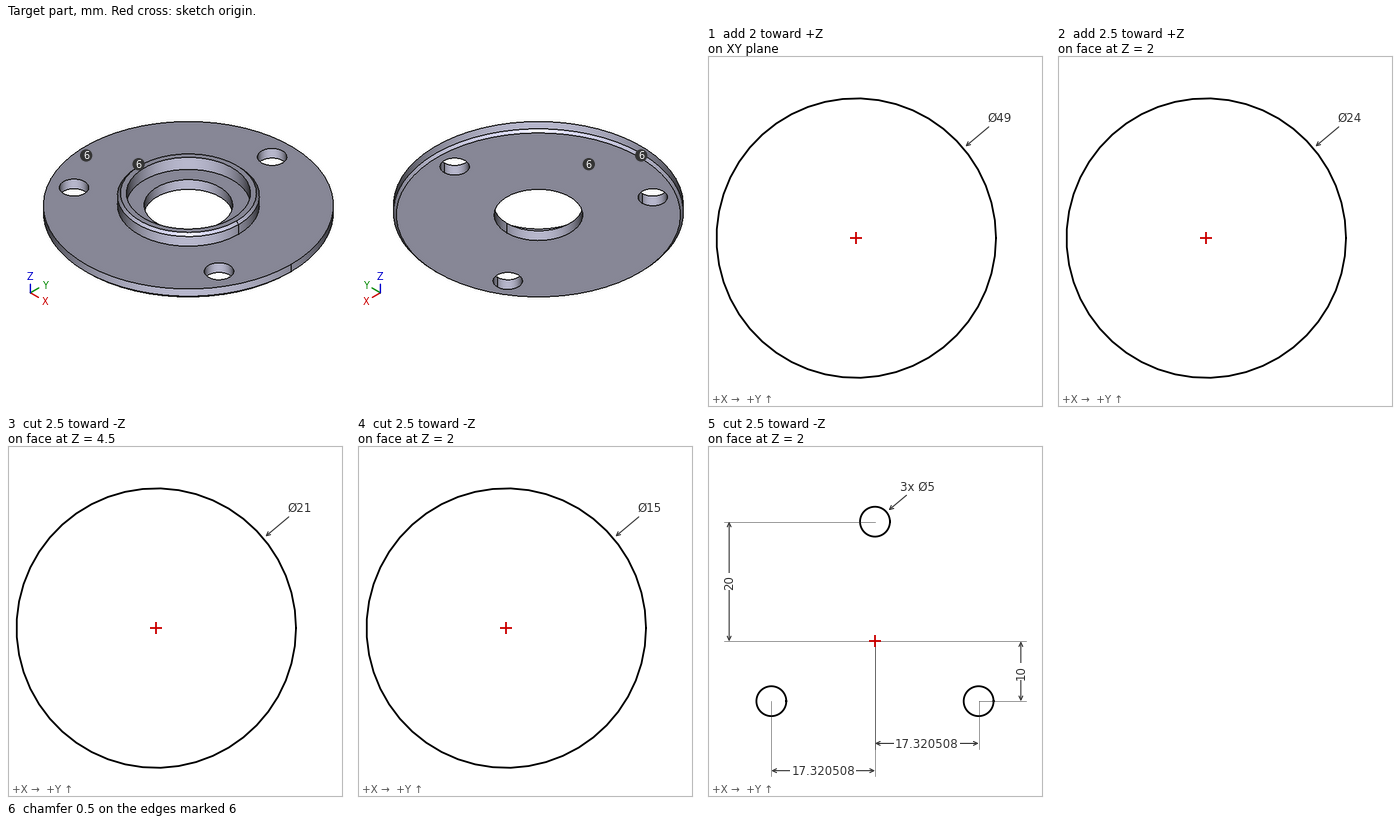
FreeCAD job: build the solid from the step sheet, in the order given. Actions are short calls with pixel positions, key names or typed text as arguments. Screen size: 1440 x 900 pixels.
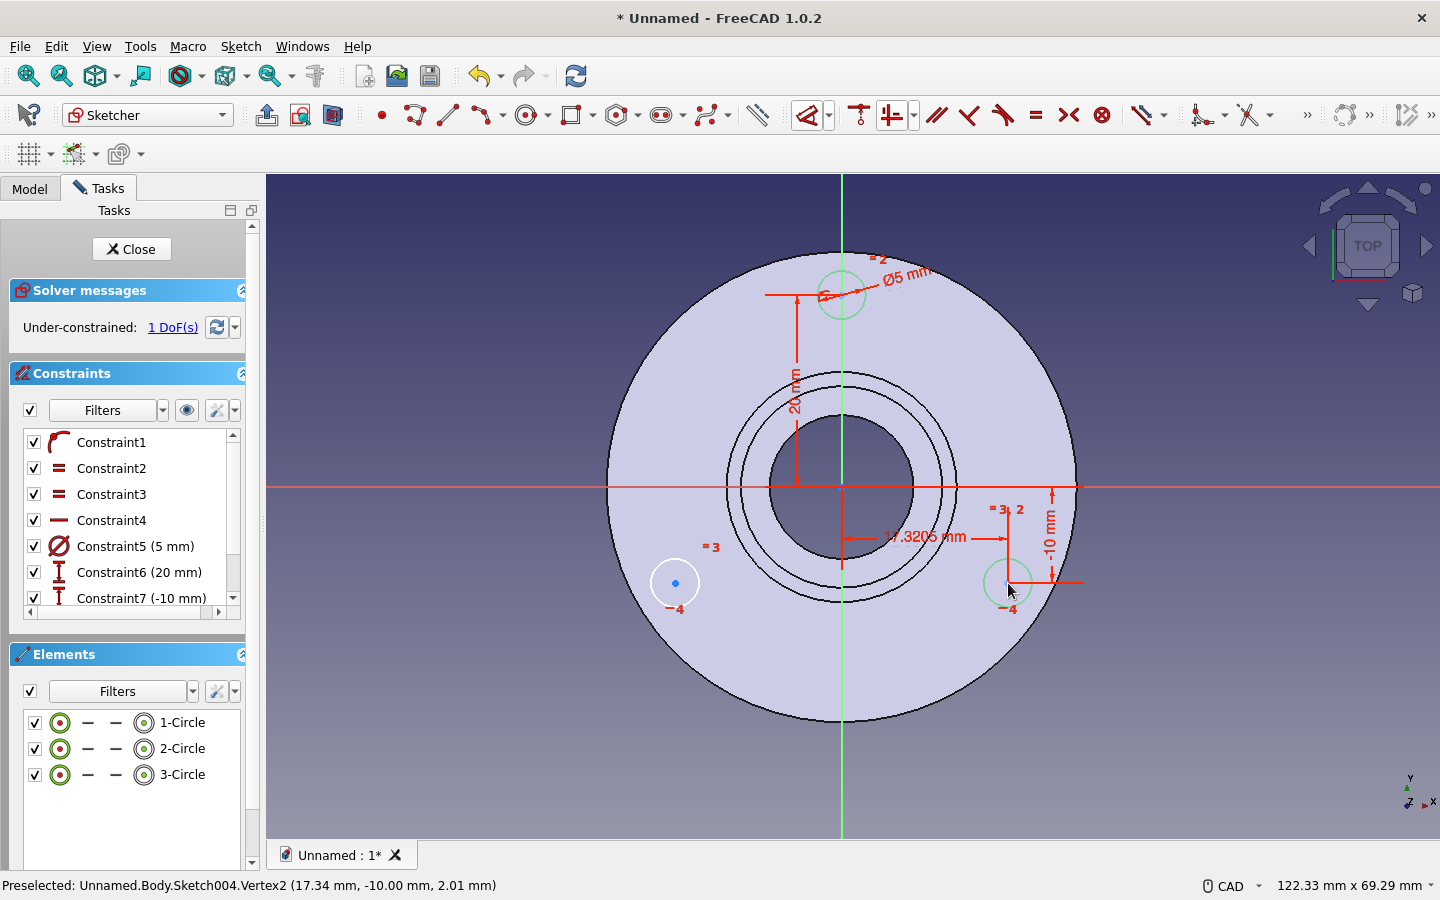
click(675, 583)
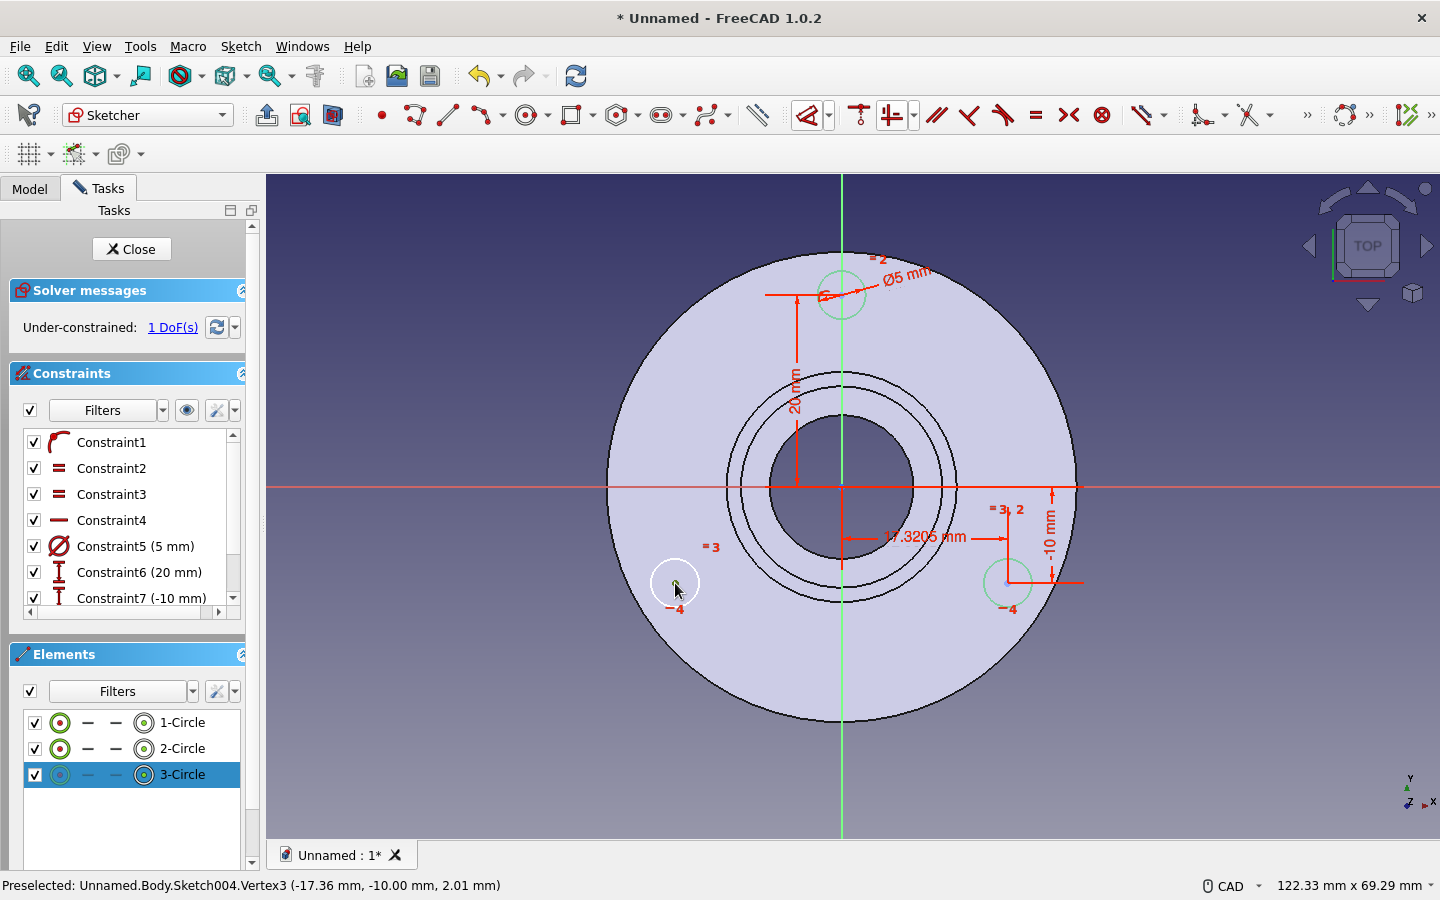
click(828, 116)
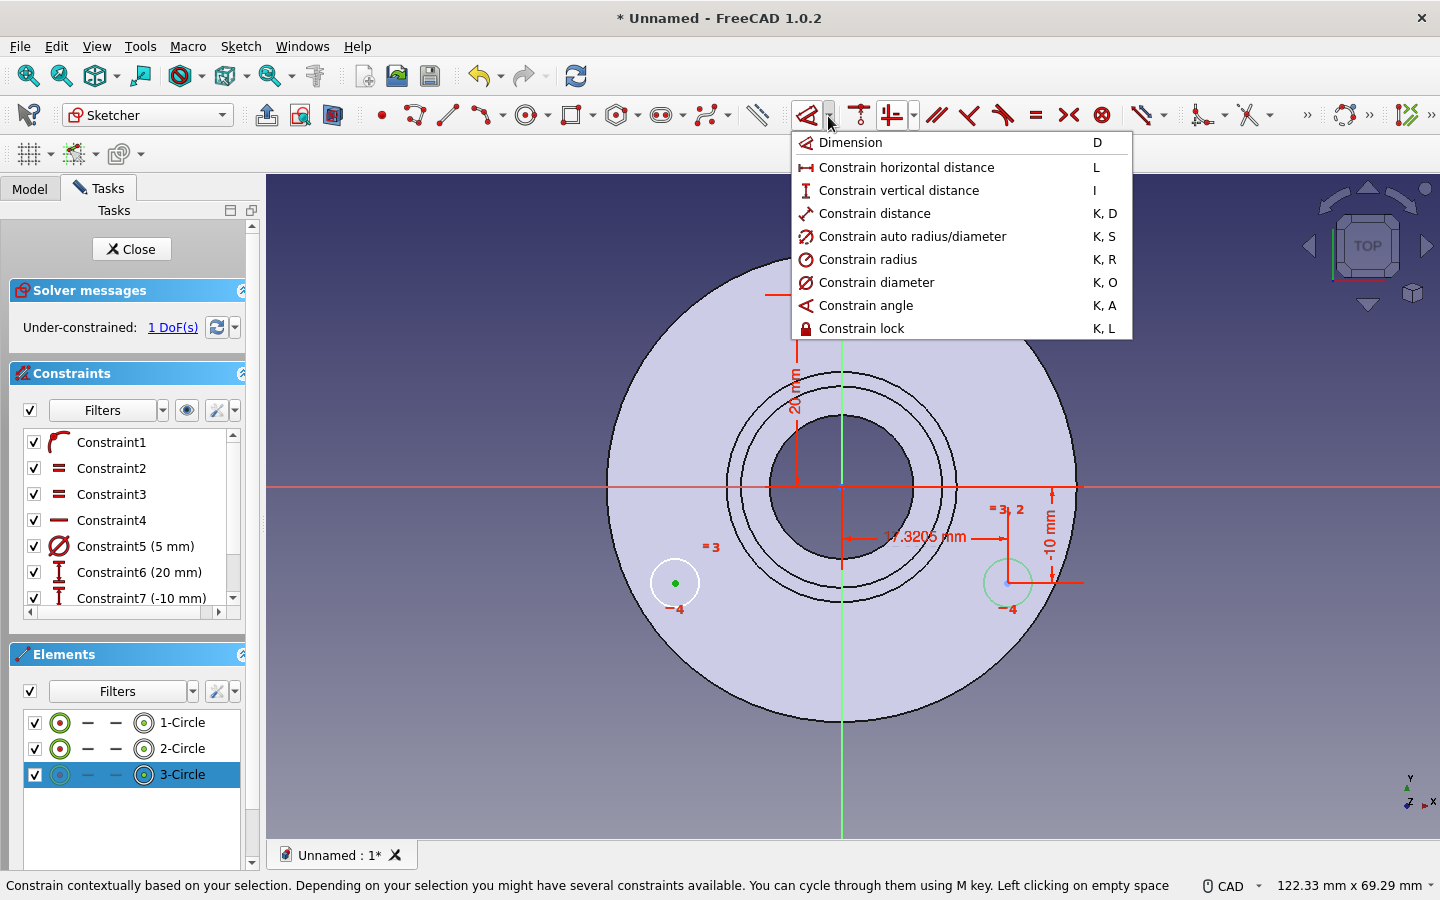
click(962, 168)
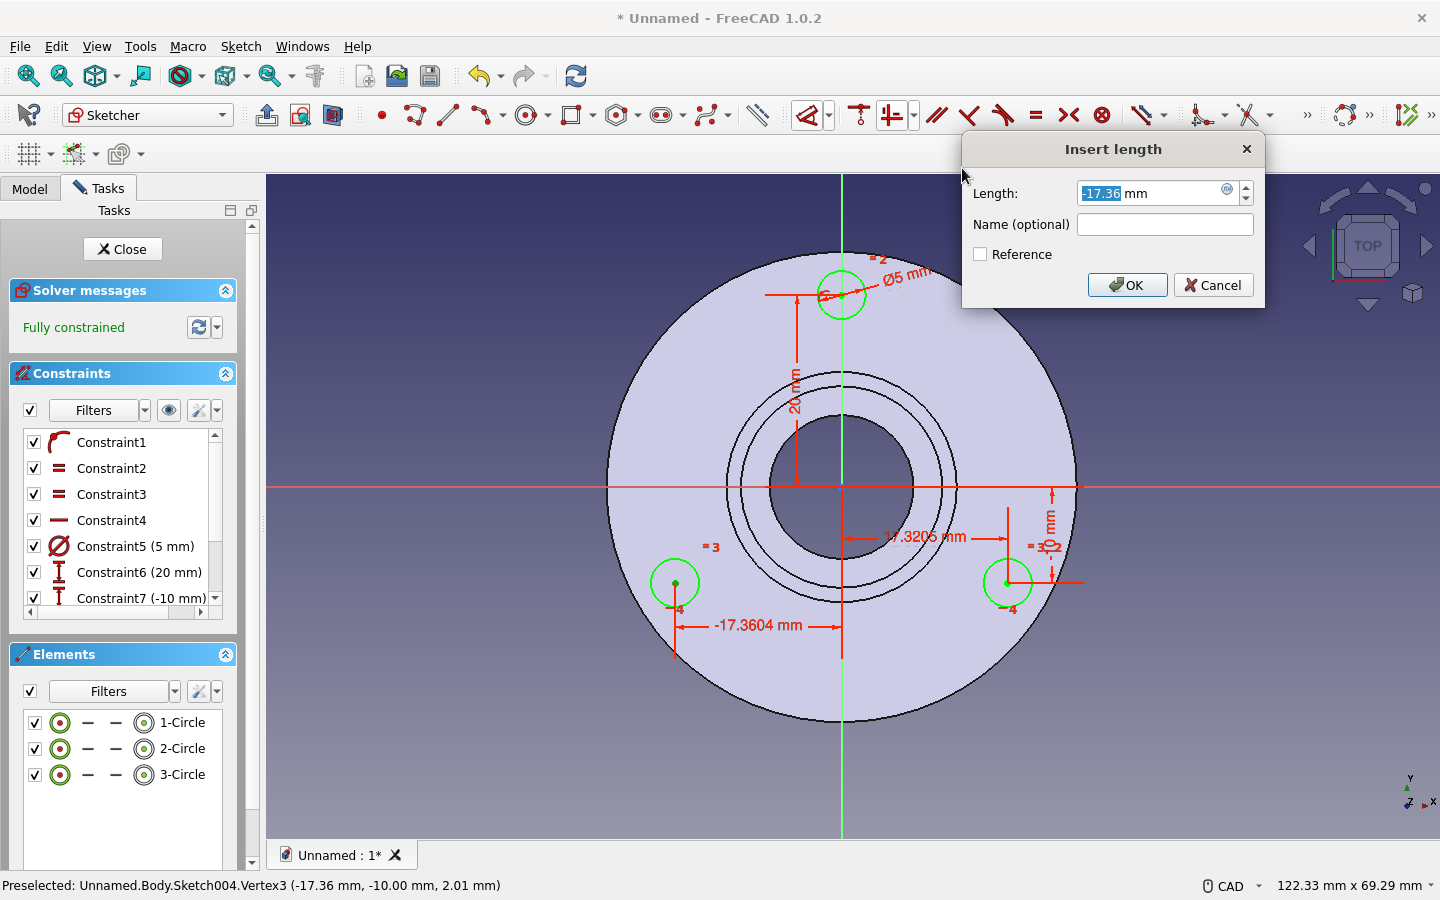
text(-17.320508)
key(Return)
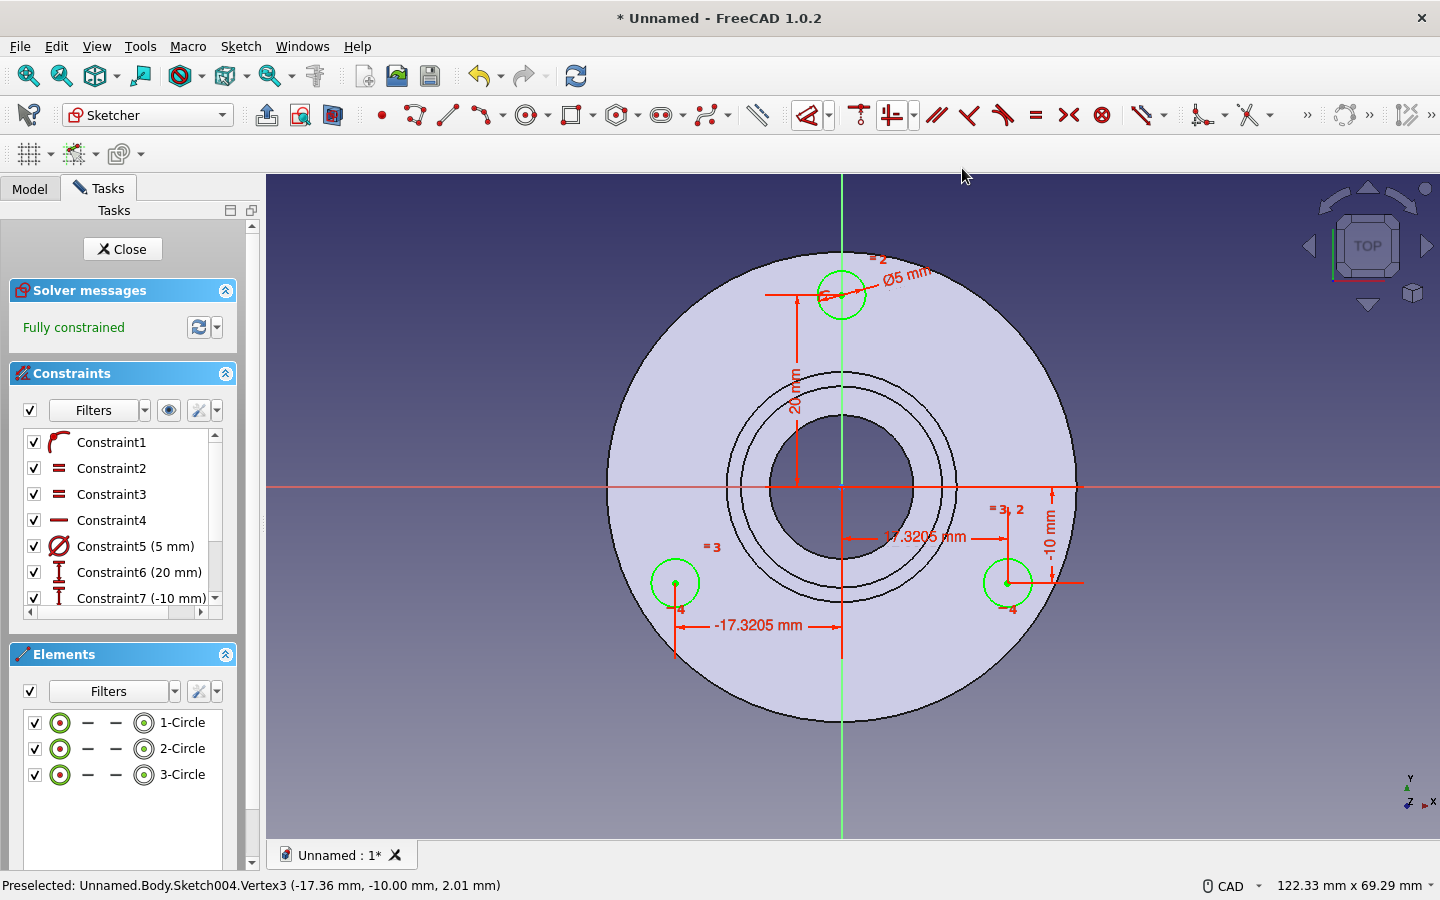
click(123, 249)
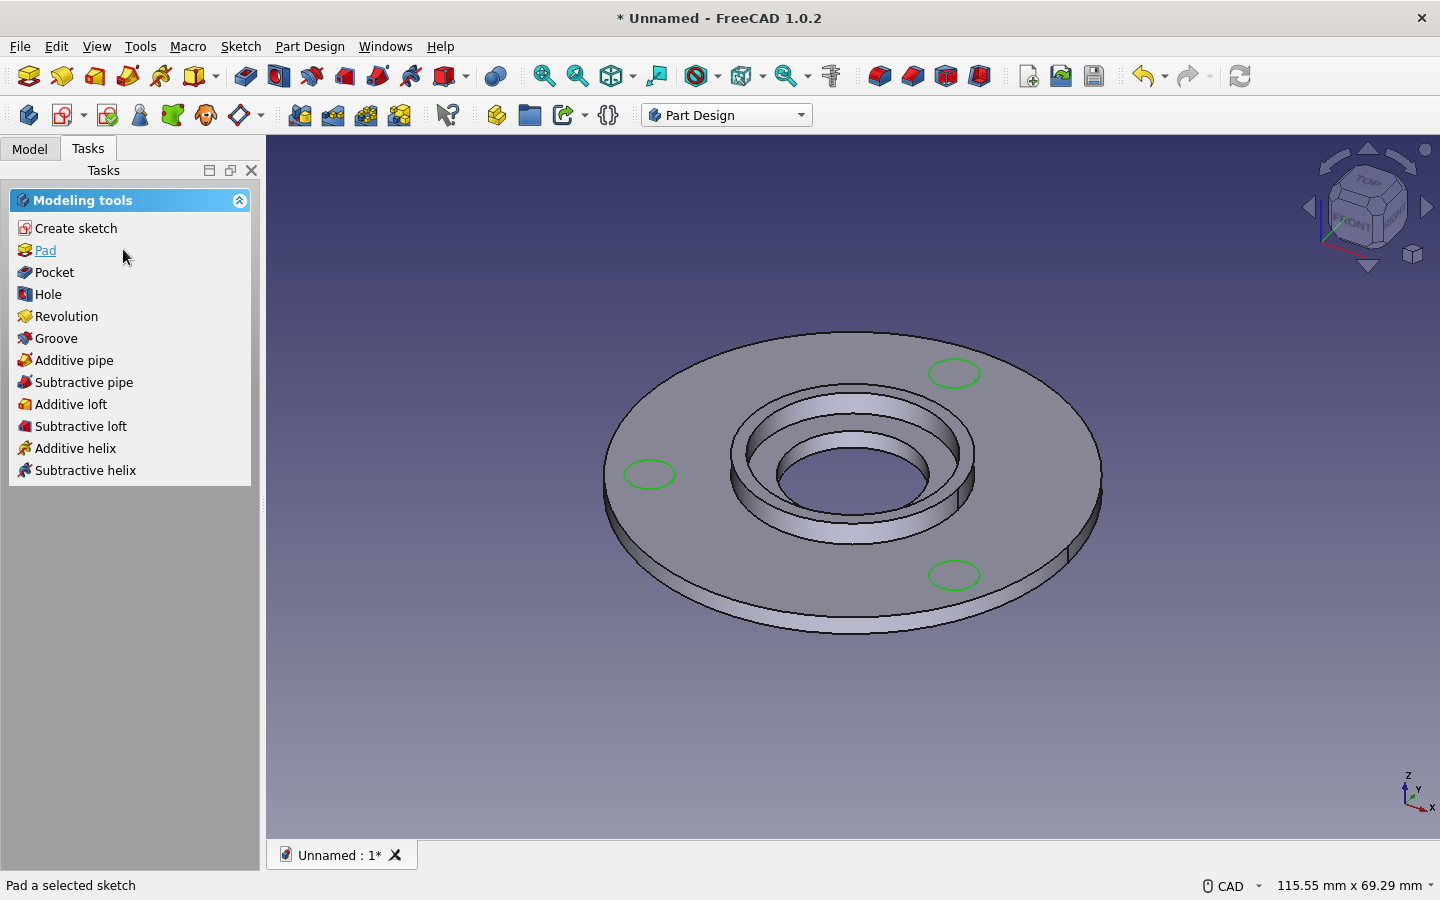
click(246, 76)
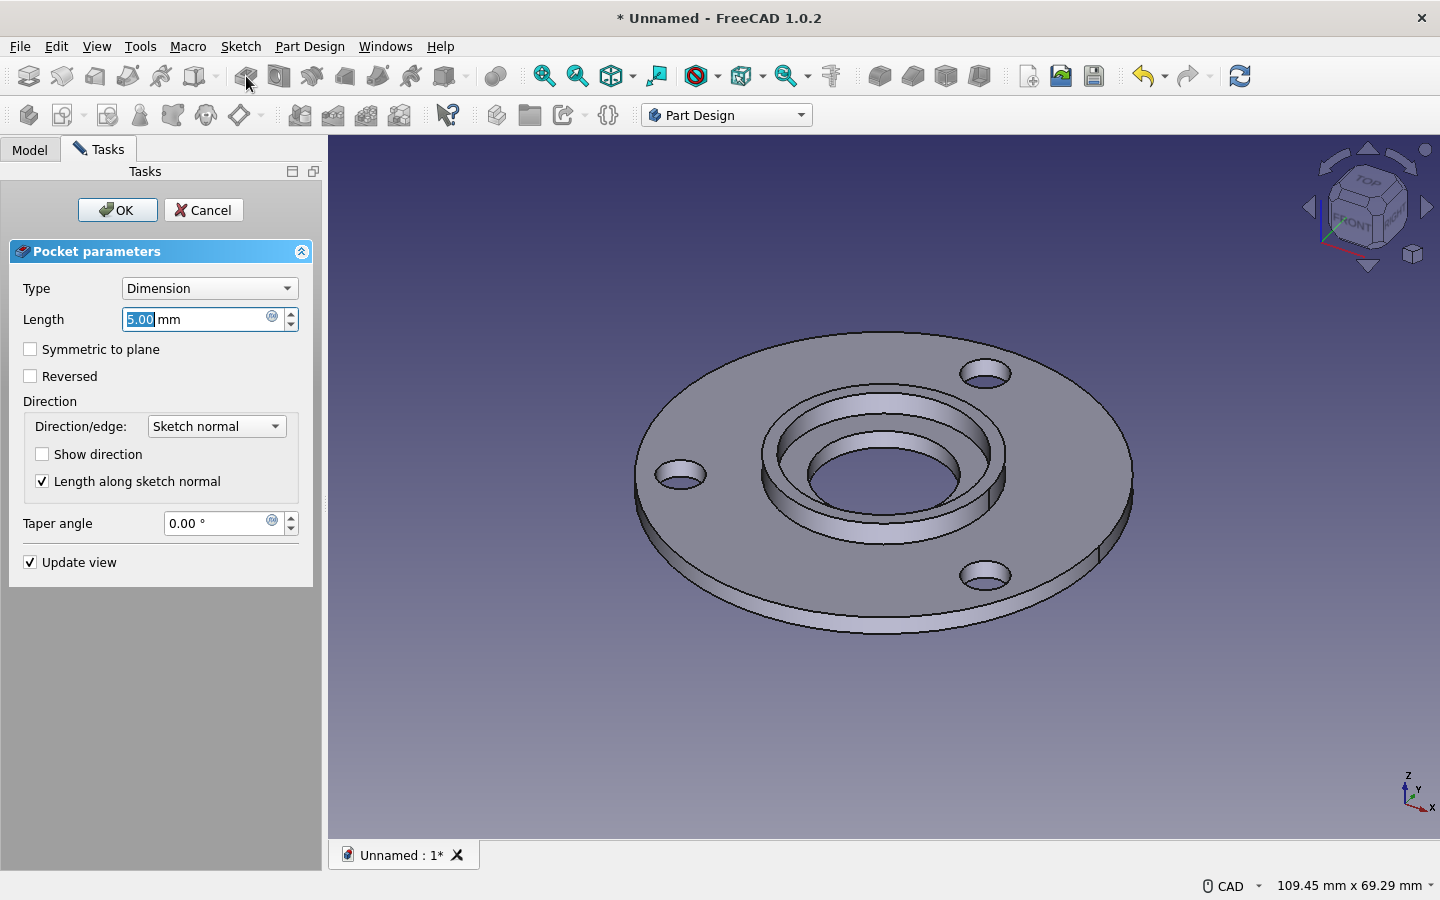
text(2.5)
key(Tab)